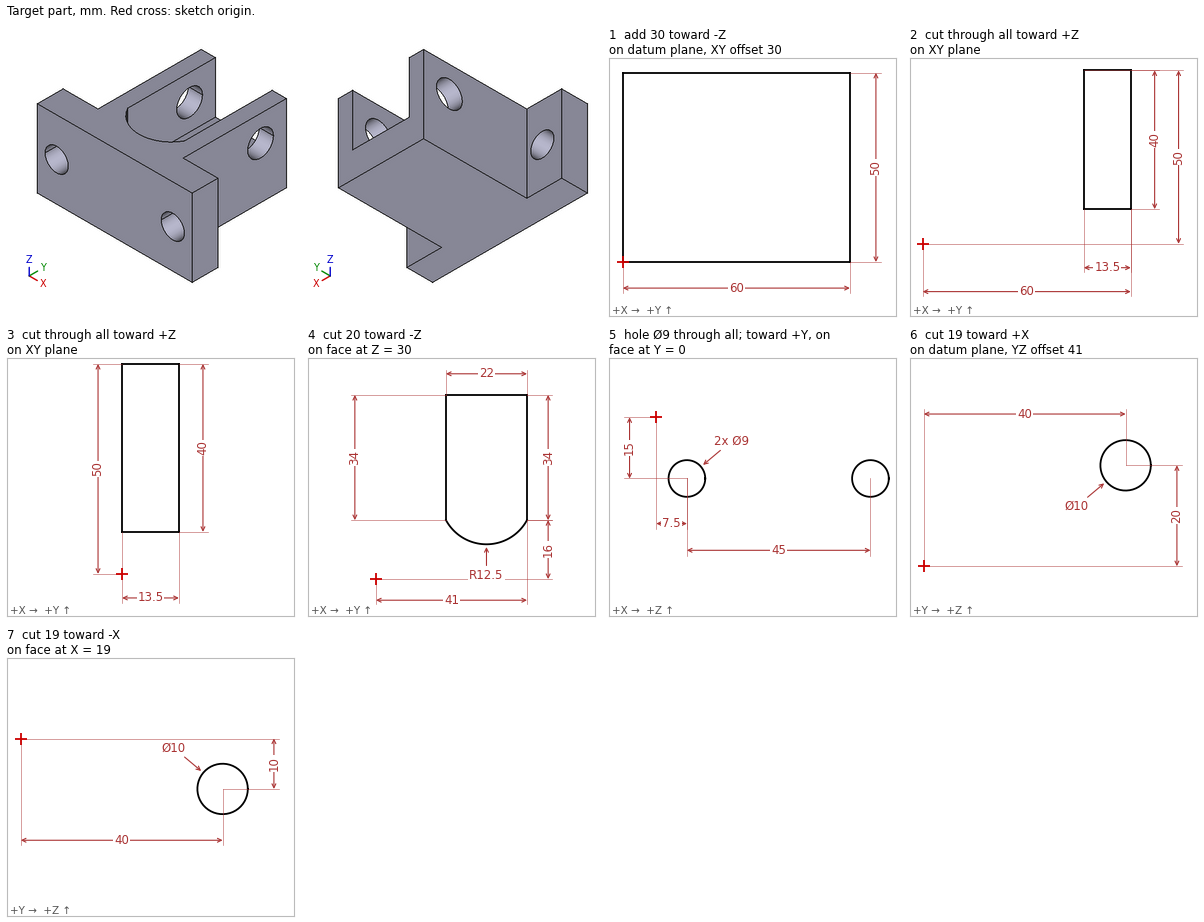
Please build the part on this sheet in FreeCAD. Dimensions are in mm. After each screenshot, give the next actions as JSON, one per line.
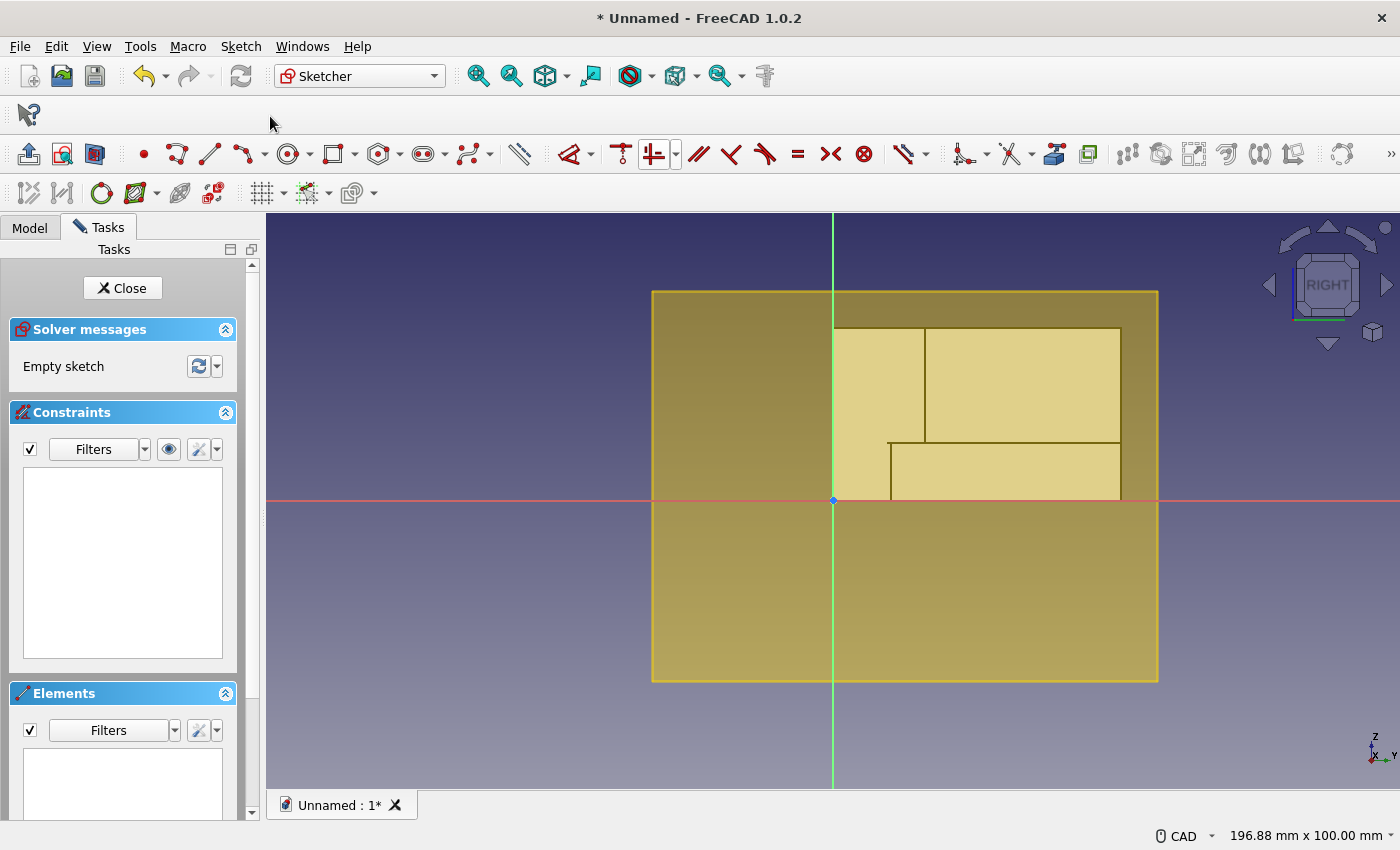
{"action": "scroll", "coordinate": [1123, 363], "scroll_direction": "up", "scroll_amount": 9}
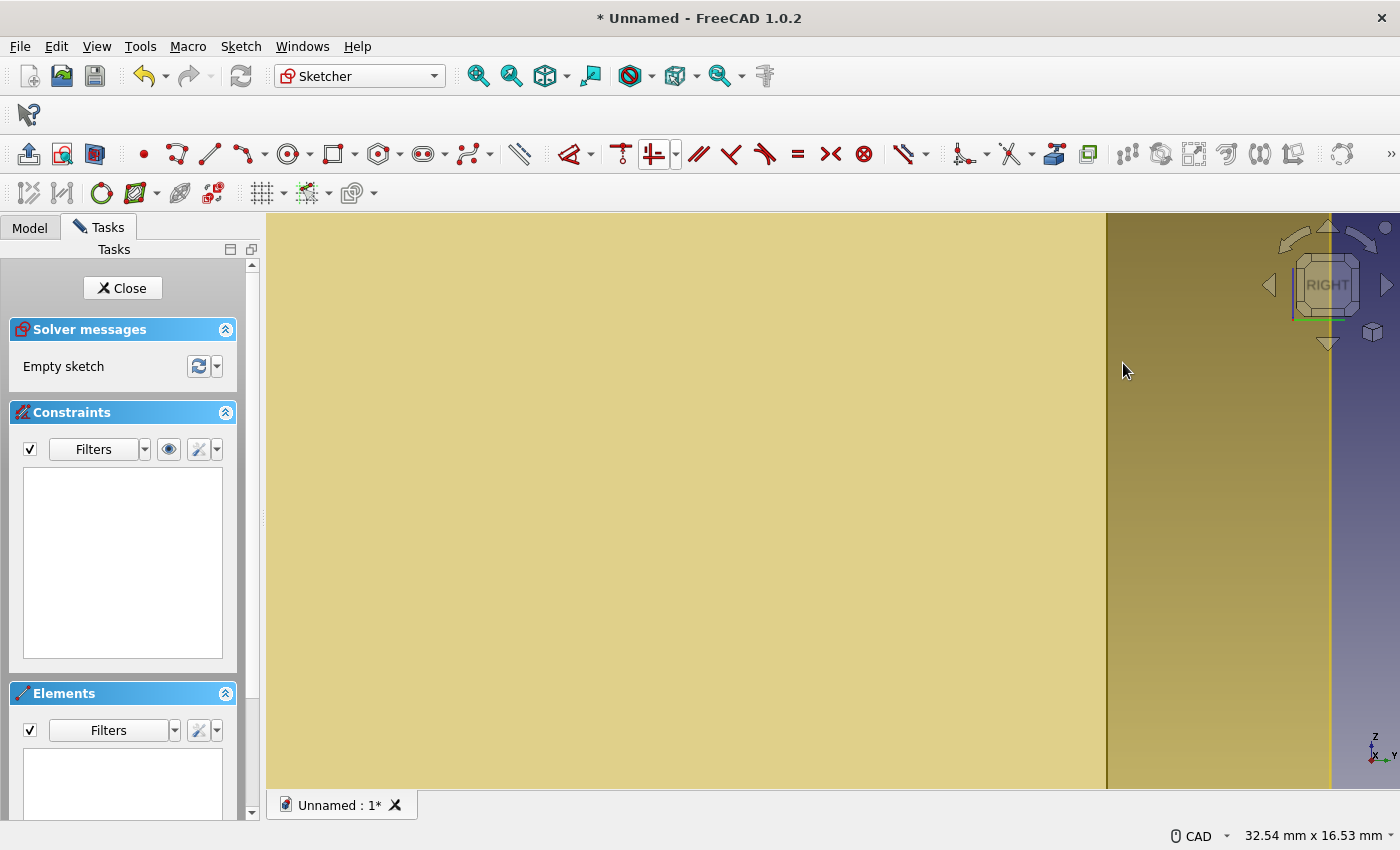
{"action": "key", "text": "g c"}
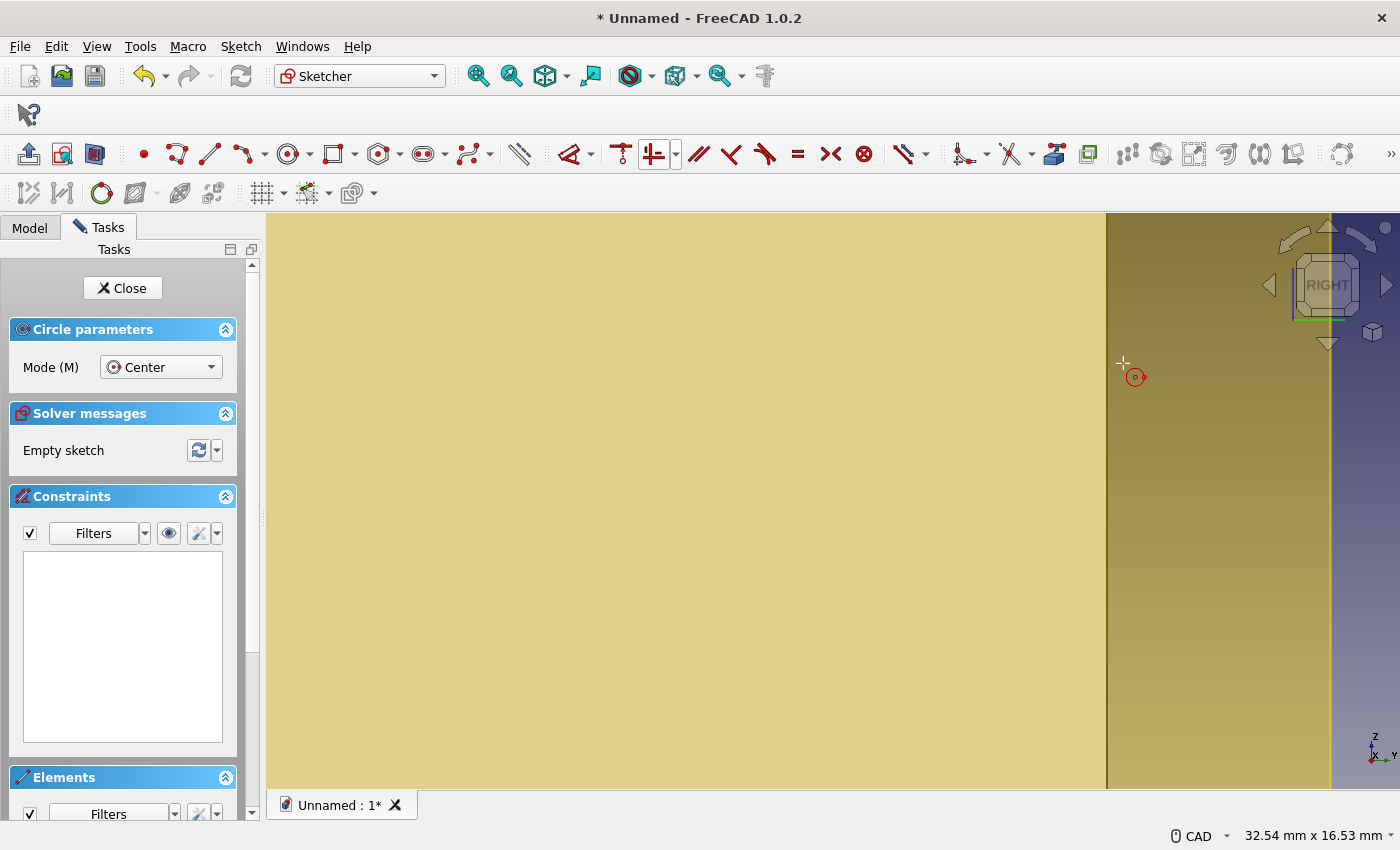
{"action": "left_click", "coordinate": [759, 500]}
{"action": "mouse_move", "coordinate": [882, 376]}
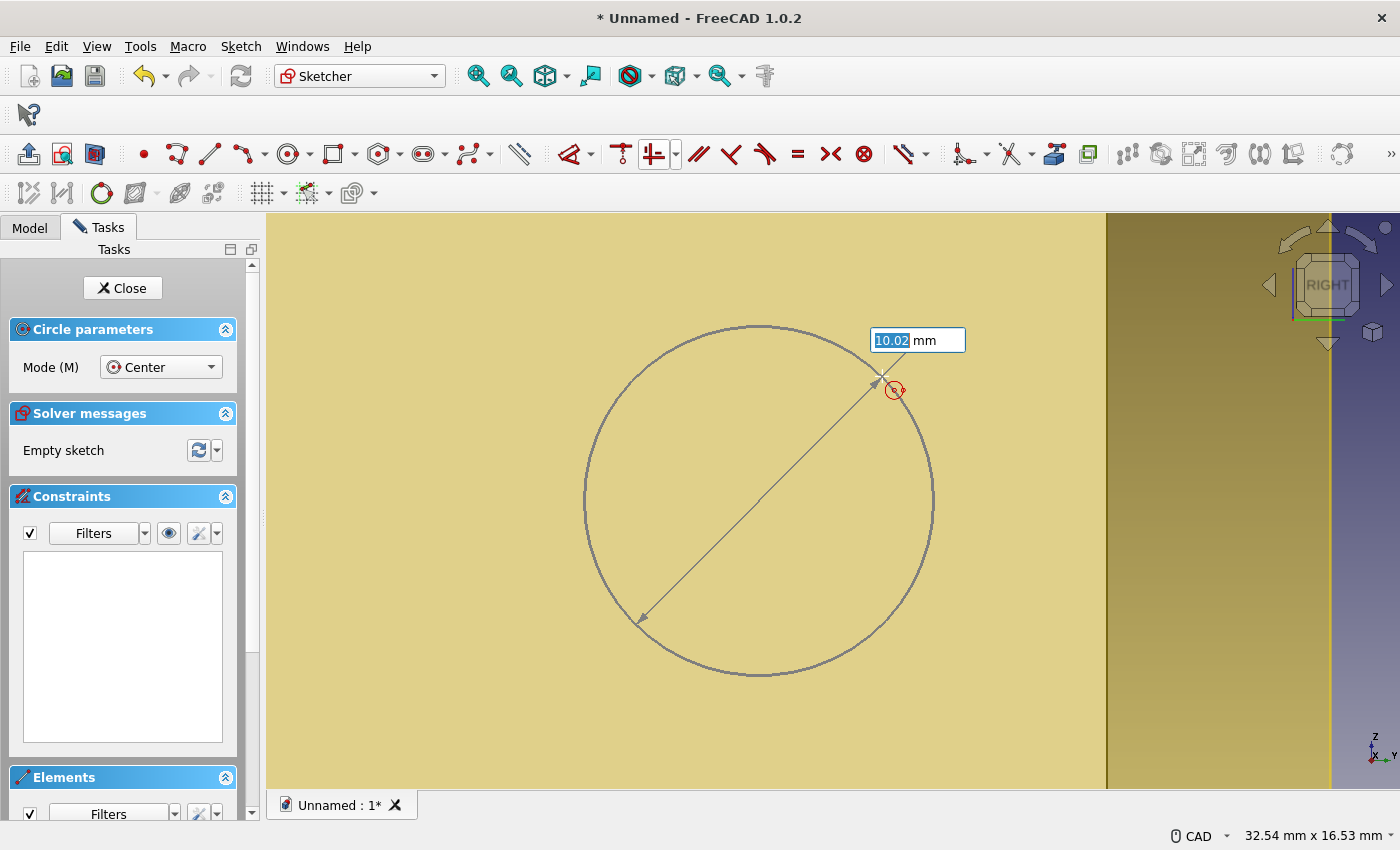
{"action": "type", "text": "10"}
{"action": "key", "text": "Return"}
{"action": "key", "text": "Escape"}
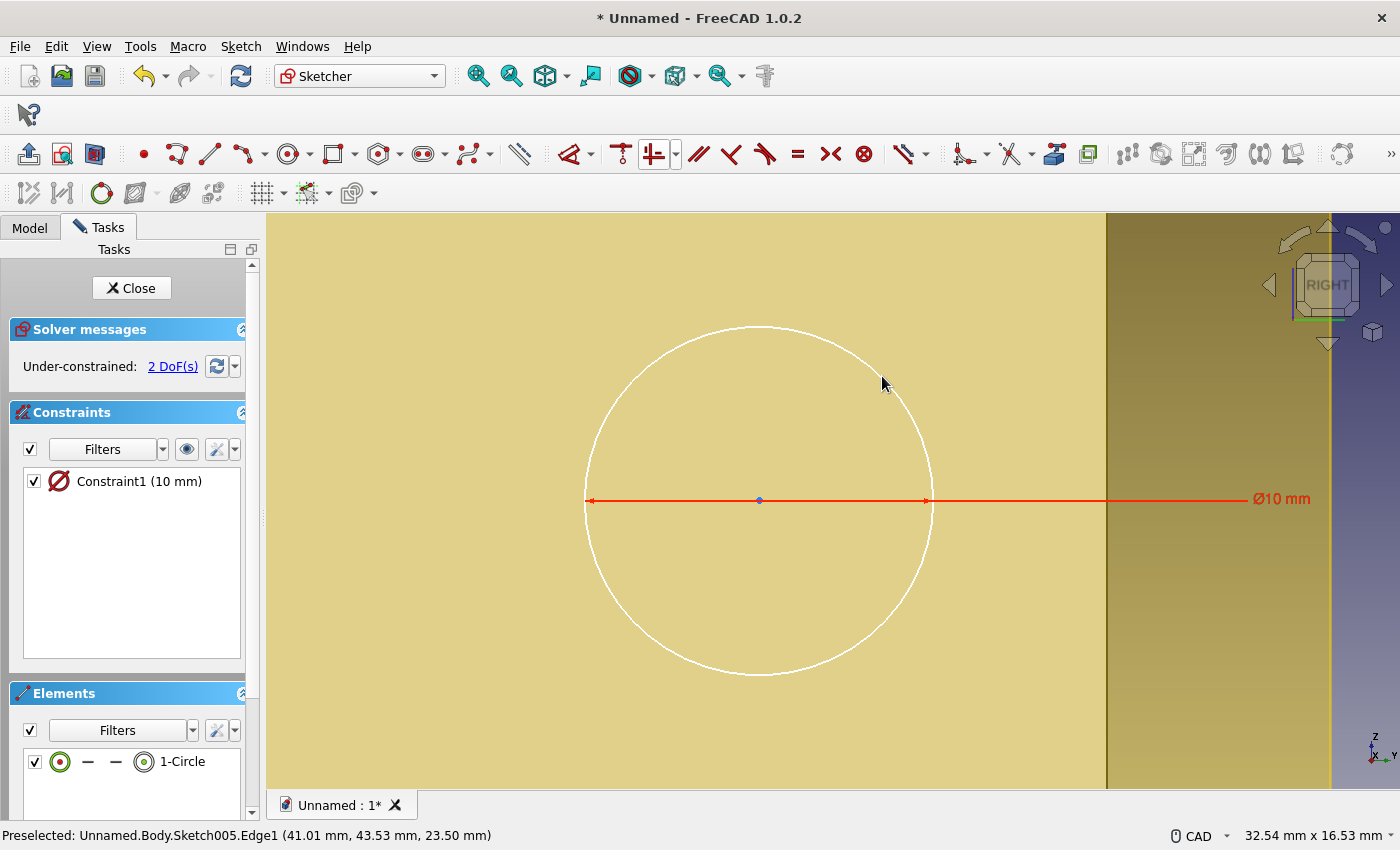
{"action": "left_click", "coordinate": [759, 501]}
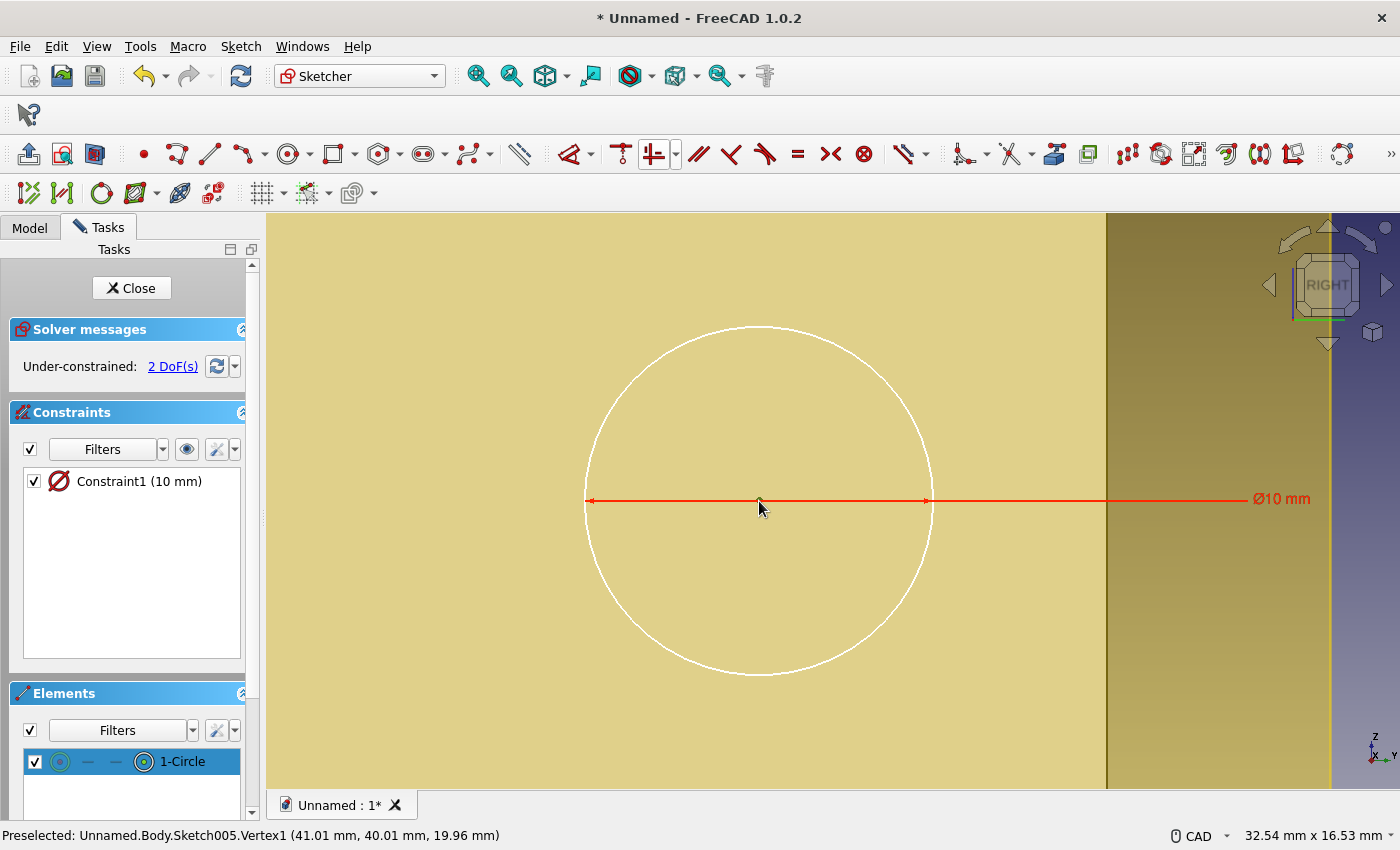
{"action": "key", "text": "l"}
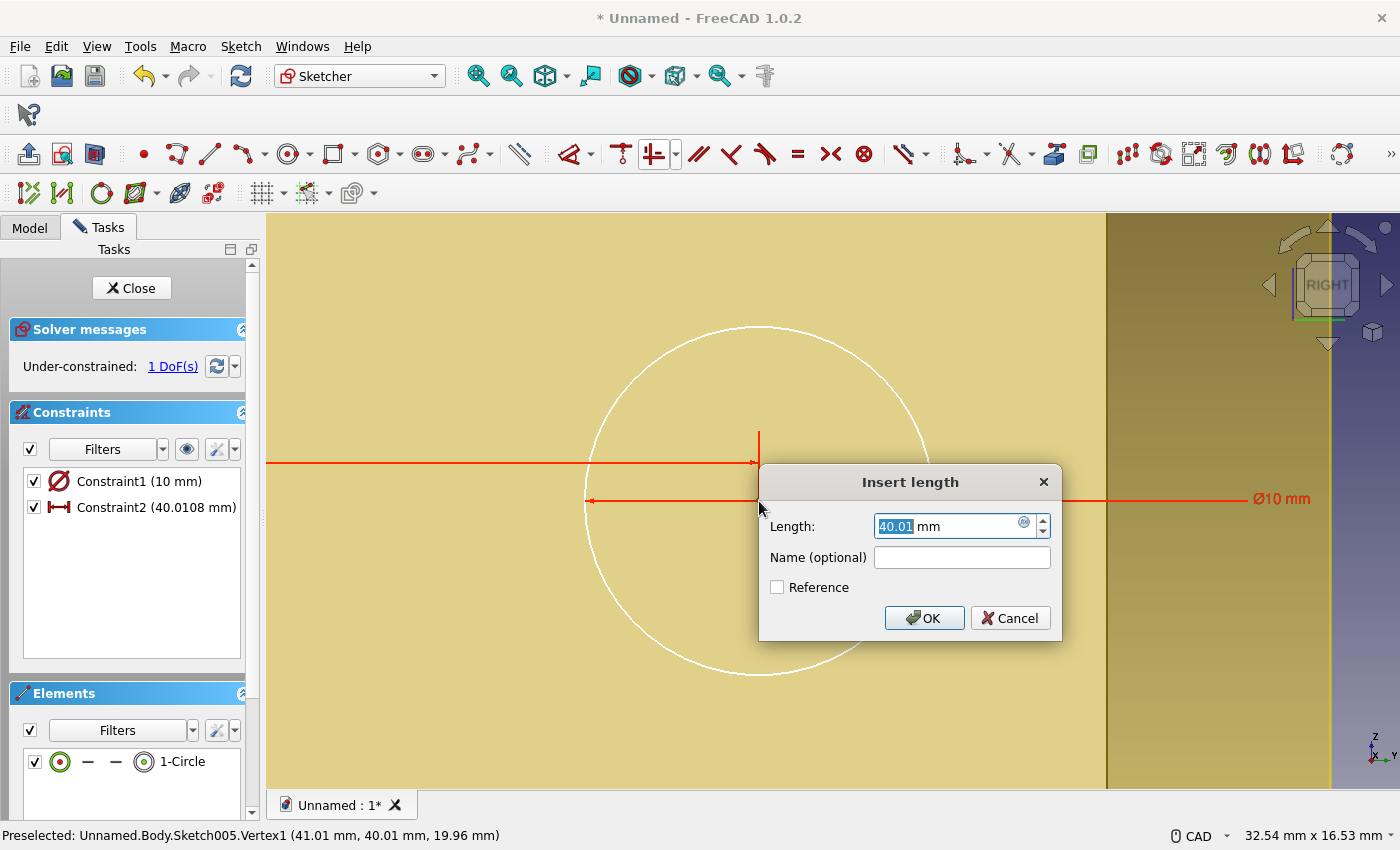
{"action": "type", "text": "40"}
{"action": "key", "text": "Return"}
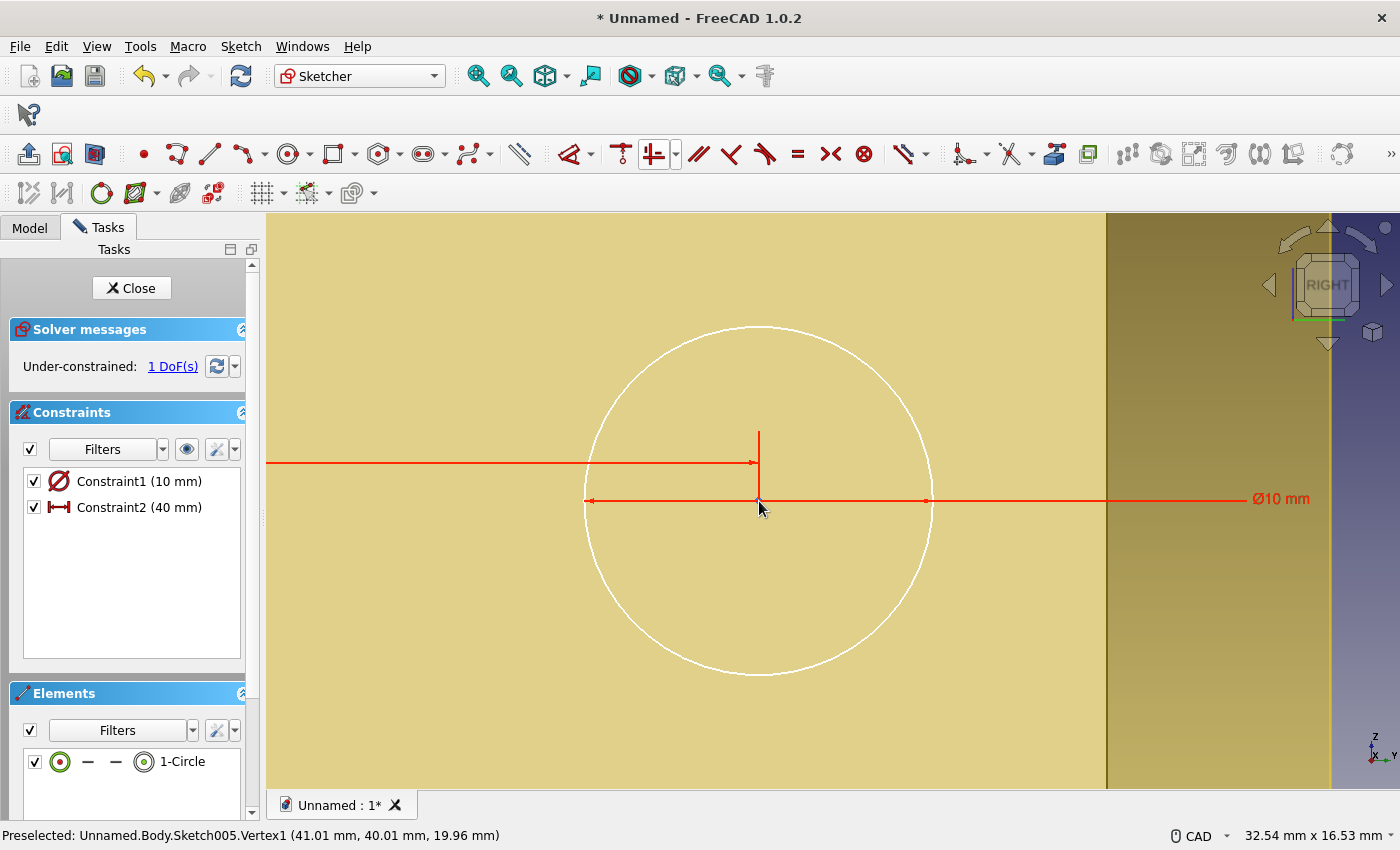
{"action": "left_click", "coordinate": [759, 501]}